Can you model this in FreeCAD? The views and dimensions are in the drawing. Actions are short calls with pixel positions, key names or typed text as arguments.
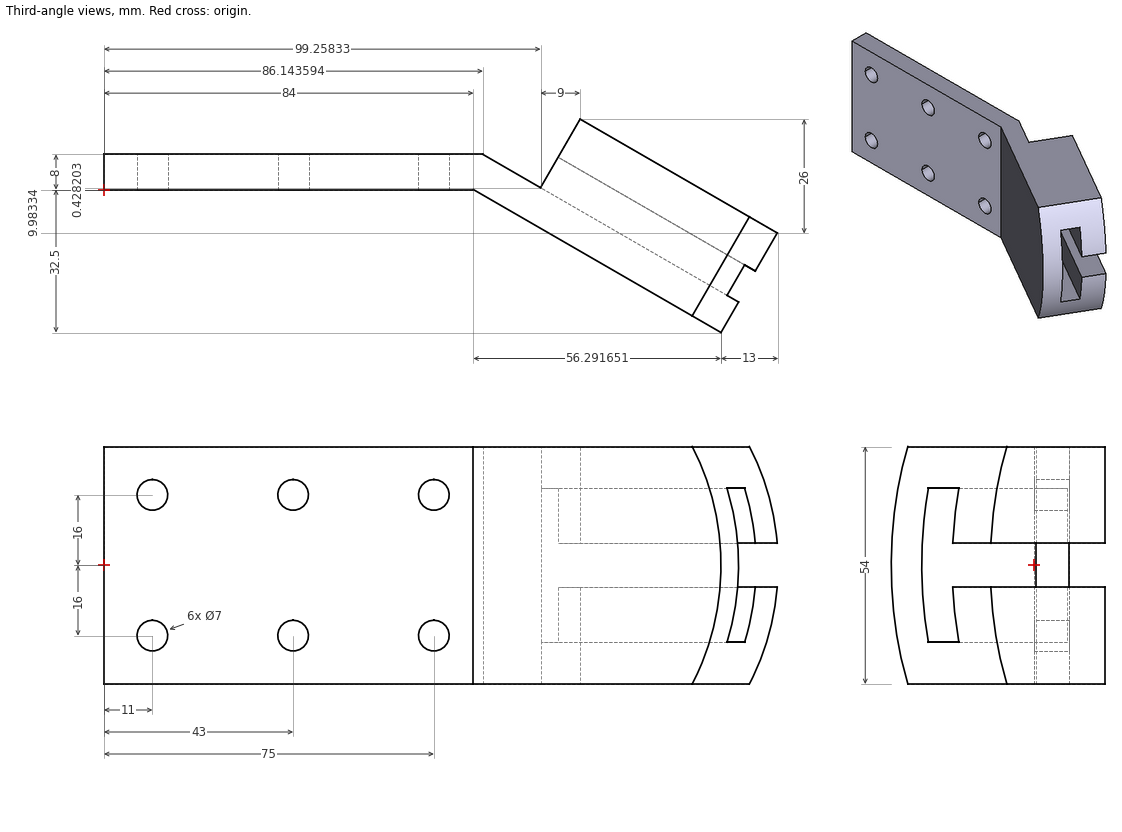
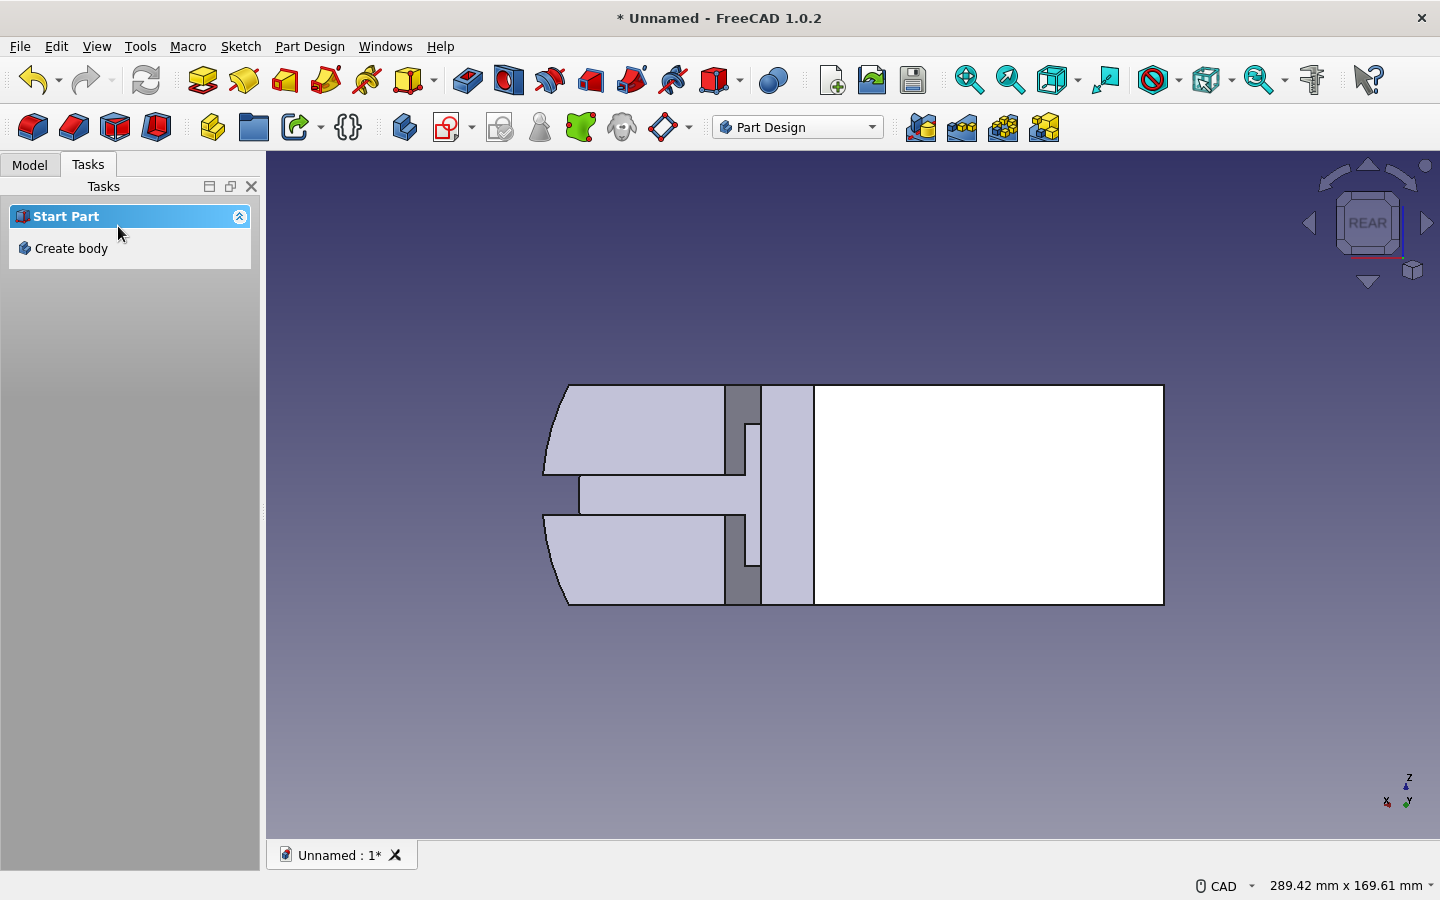
click(939, 494)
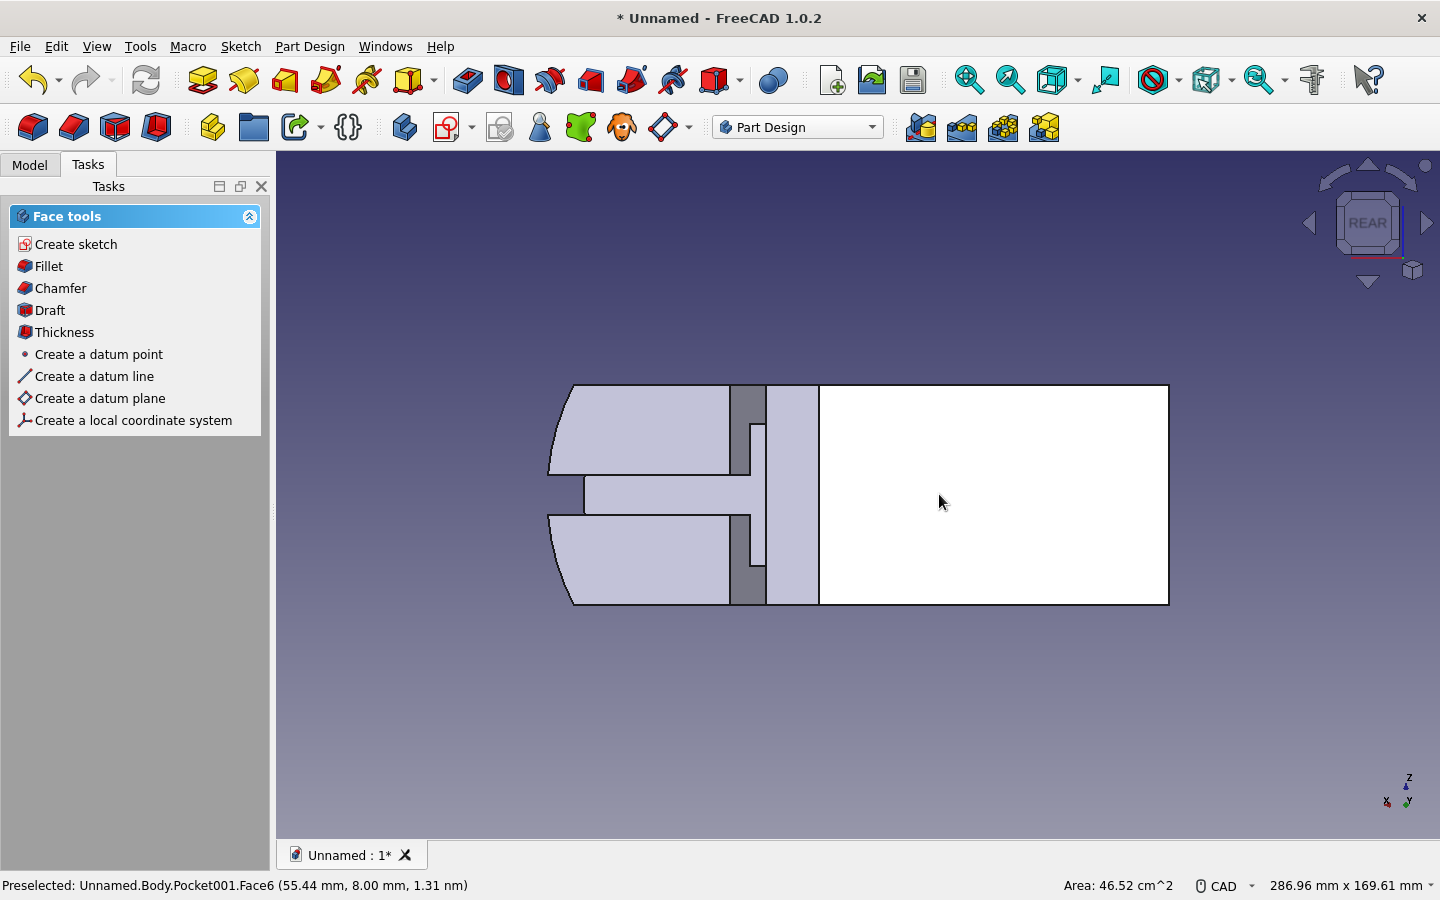
click(446, 128)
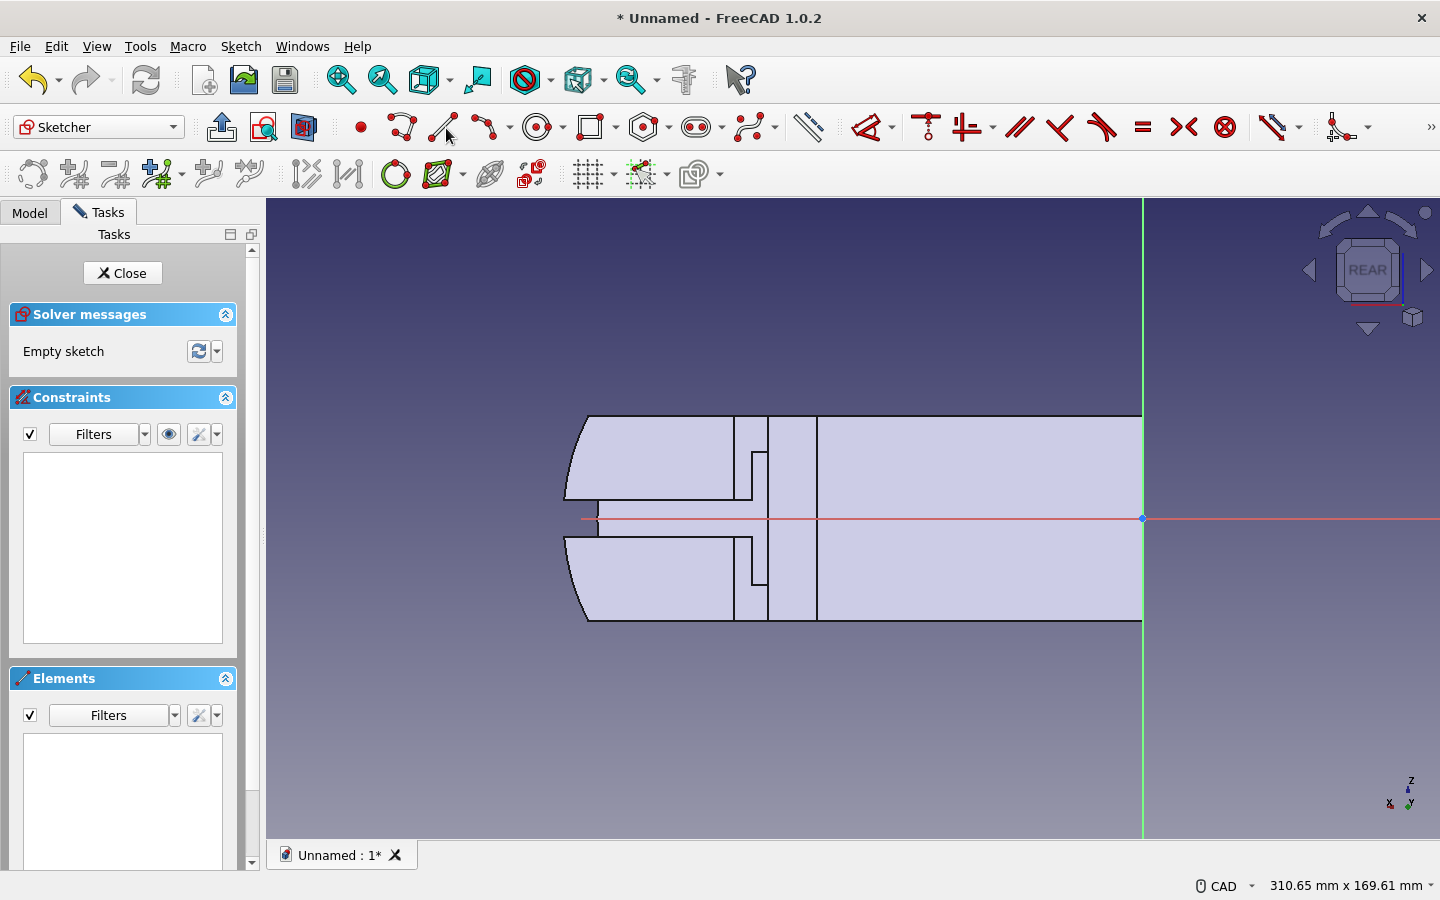
scroll(1166, 519, up, 4)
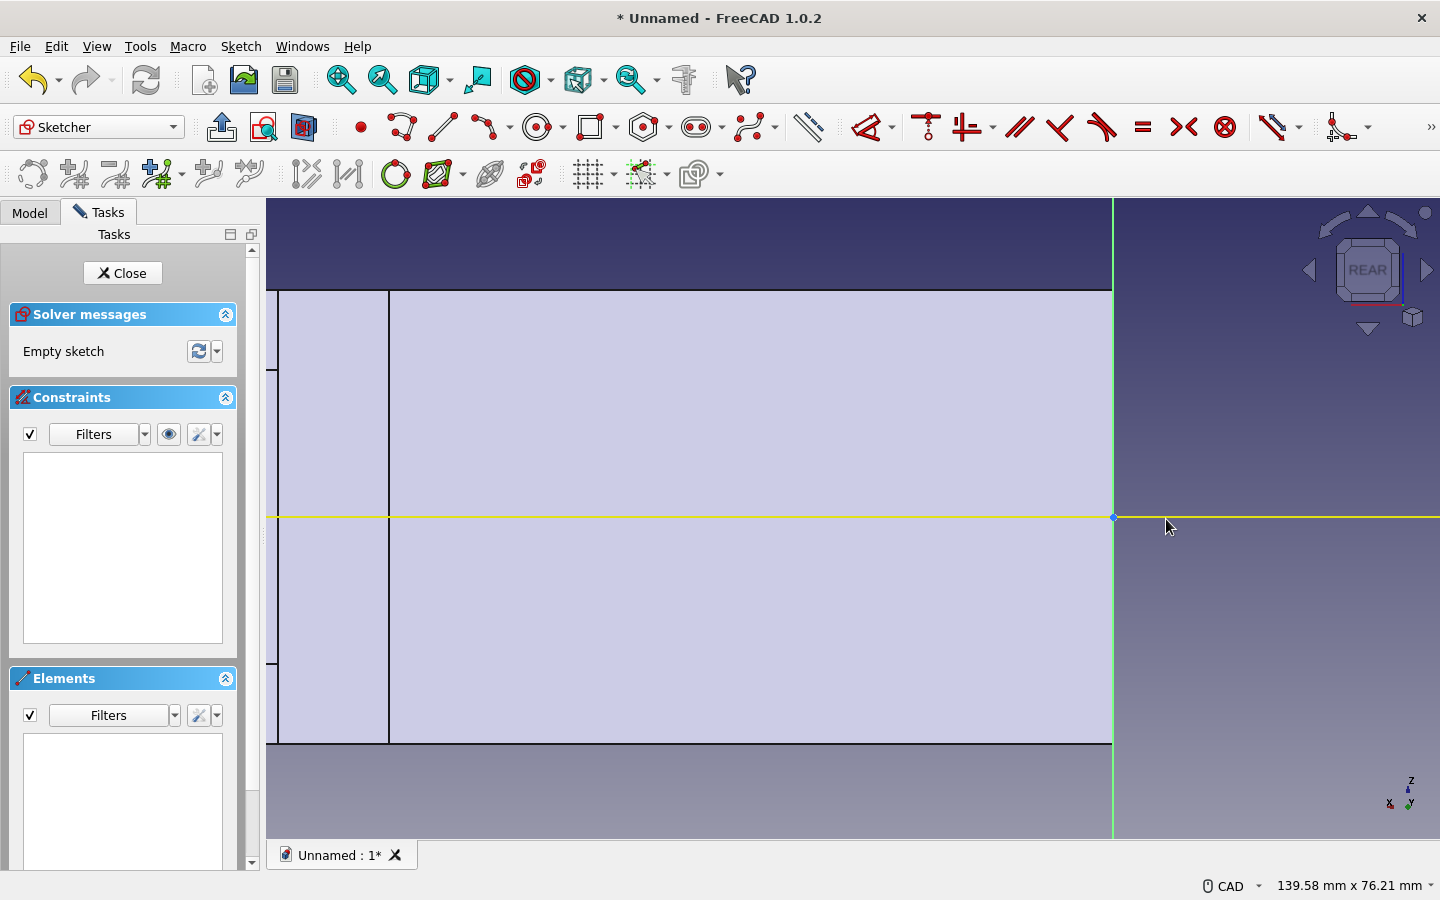
key(g)
key(c)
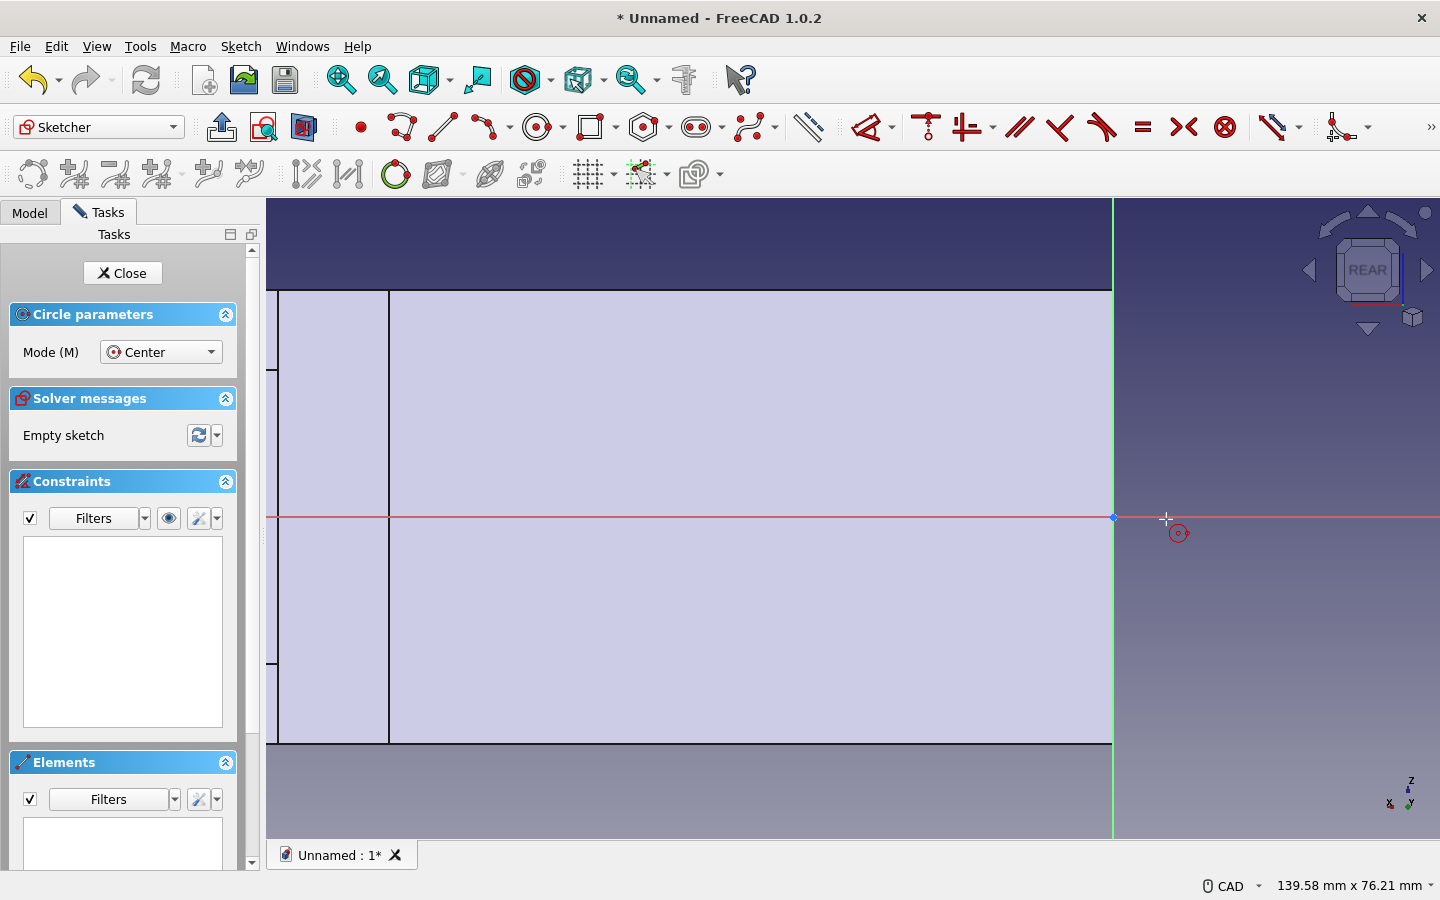
click(1021, 652)
move(1041, 631)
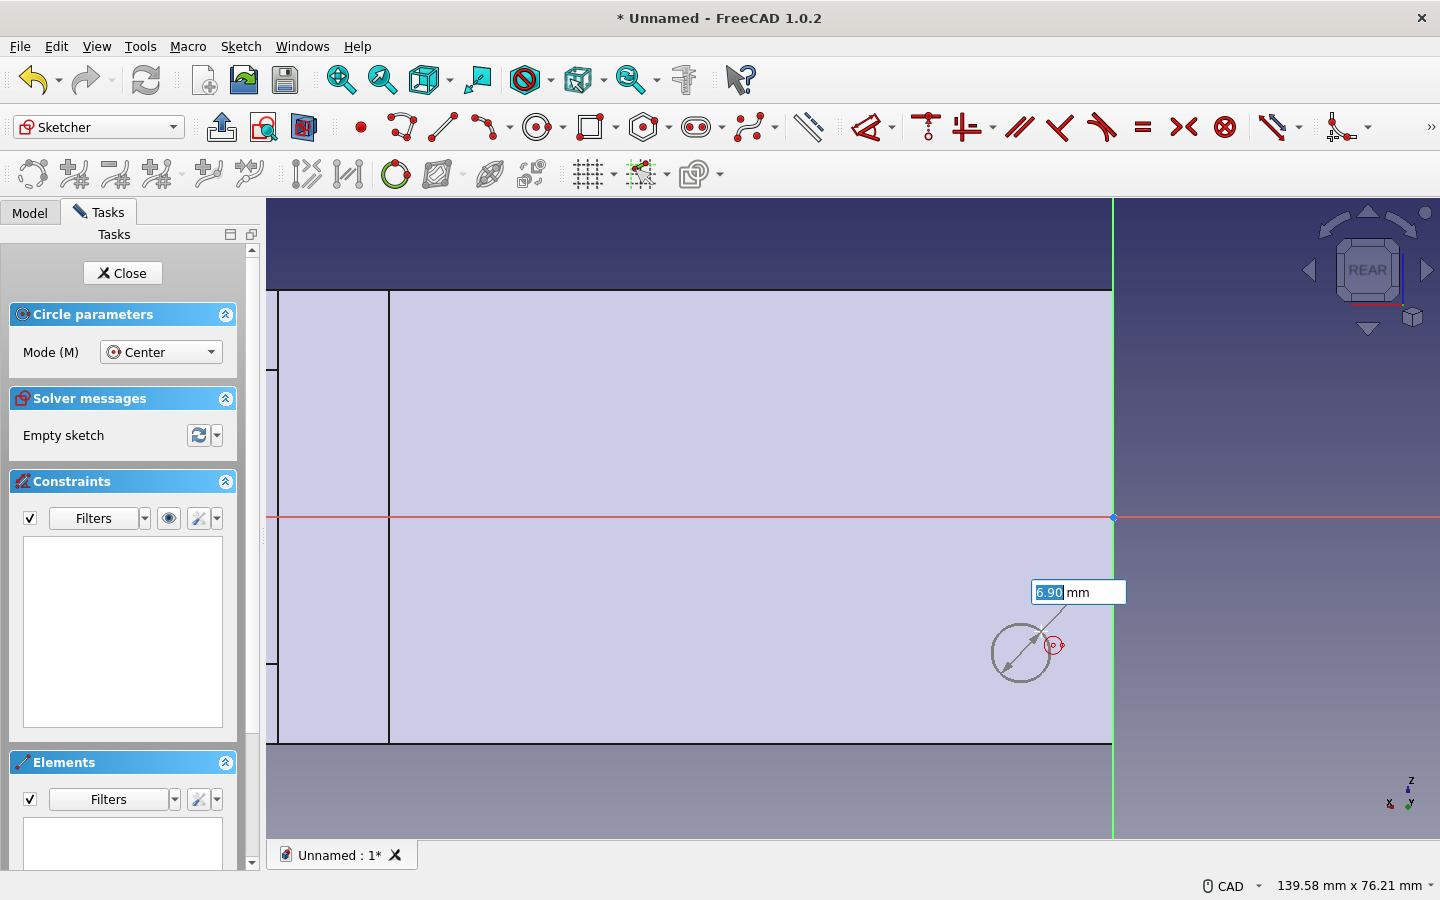
text(7)
key(Return)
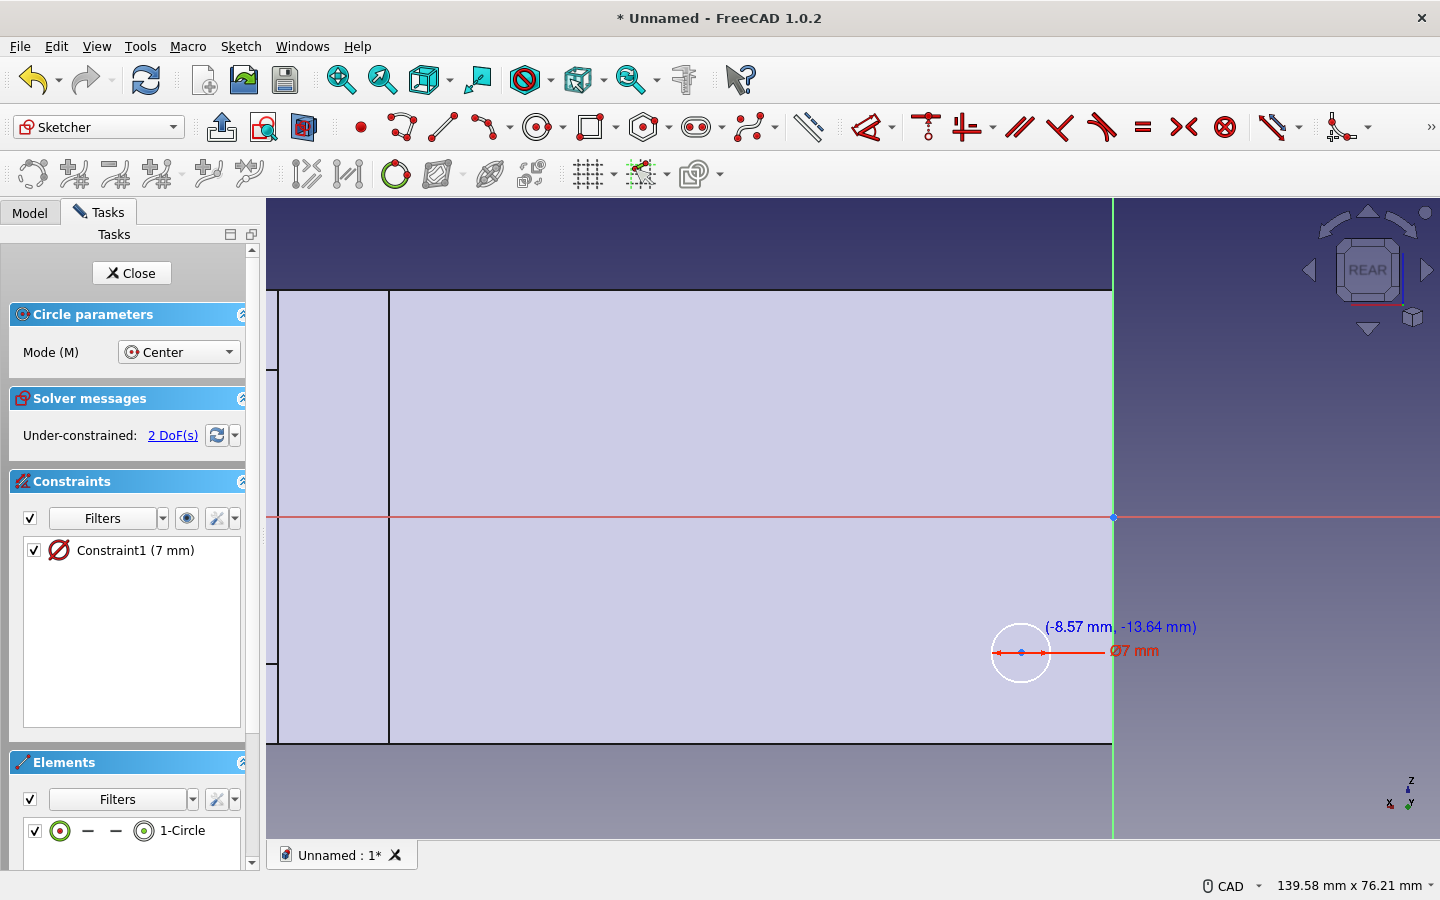
click(751, 652)
move(772, 631)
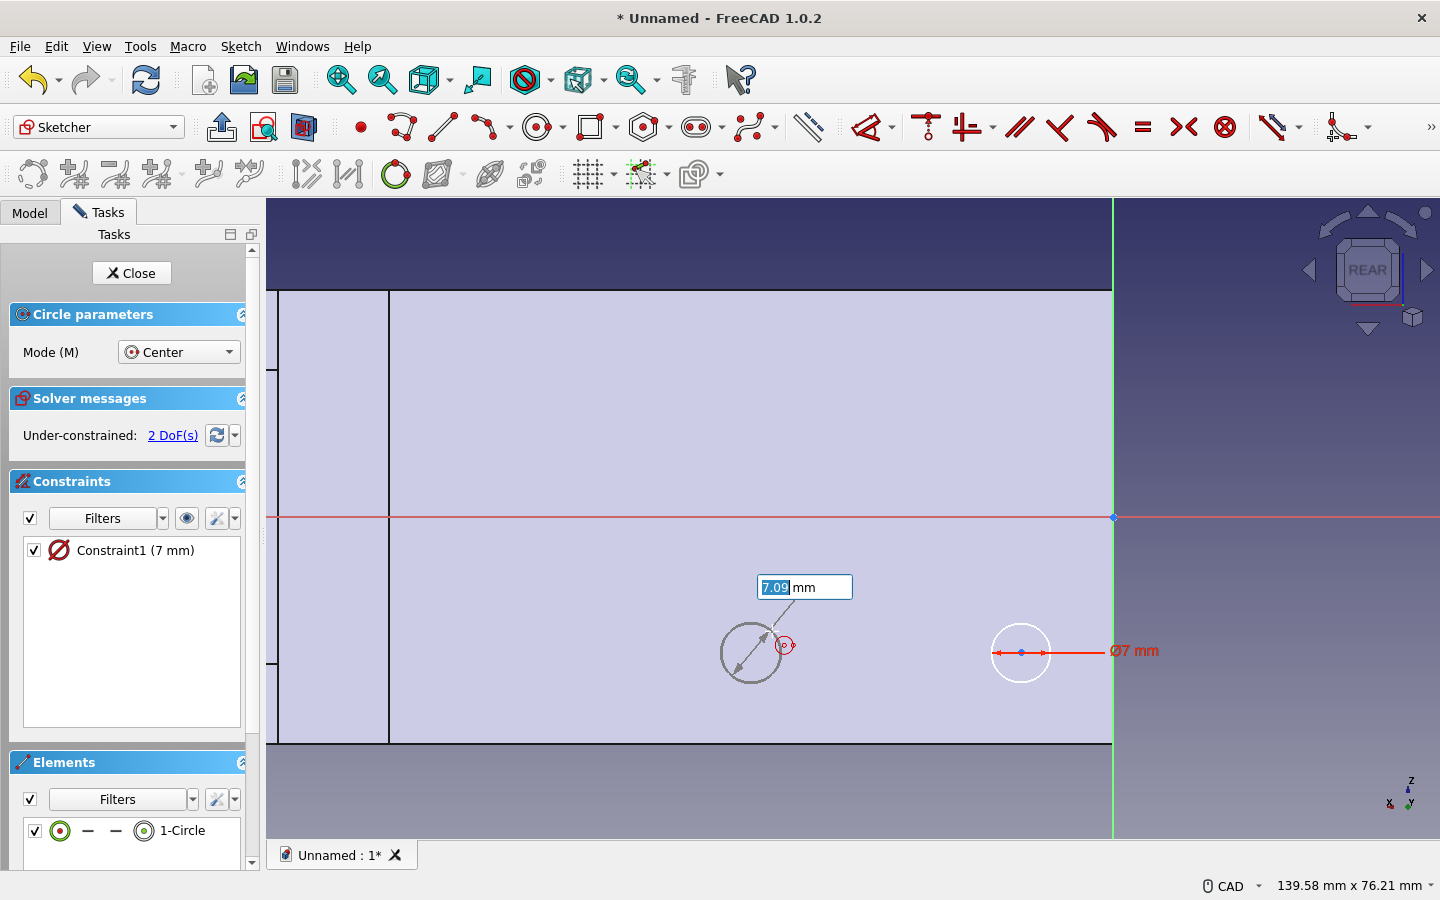
text(7)
key(Return)